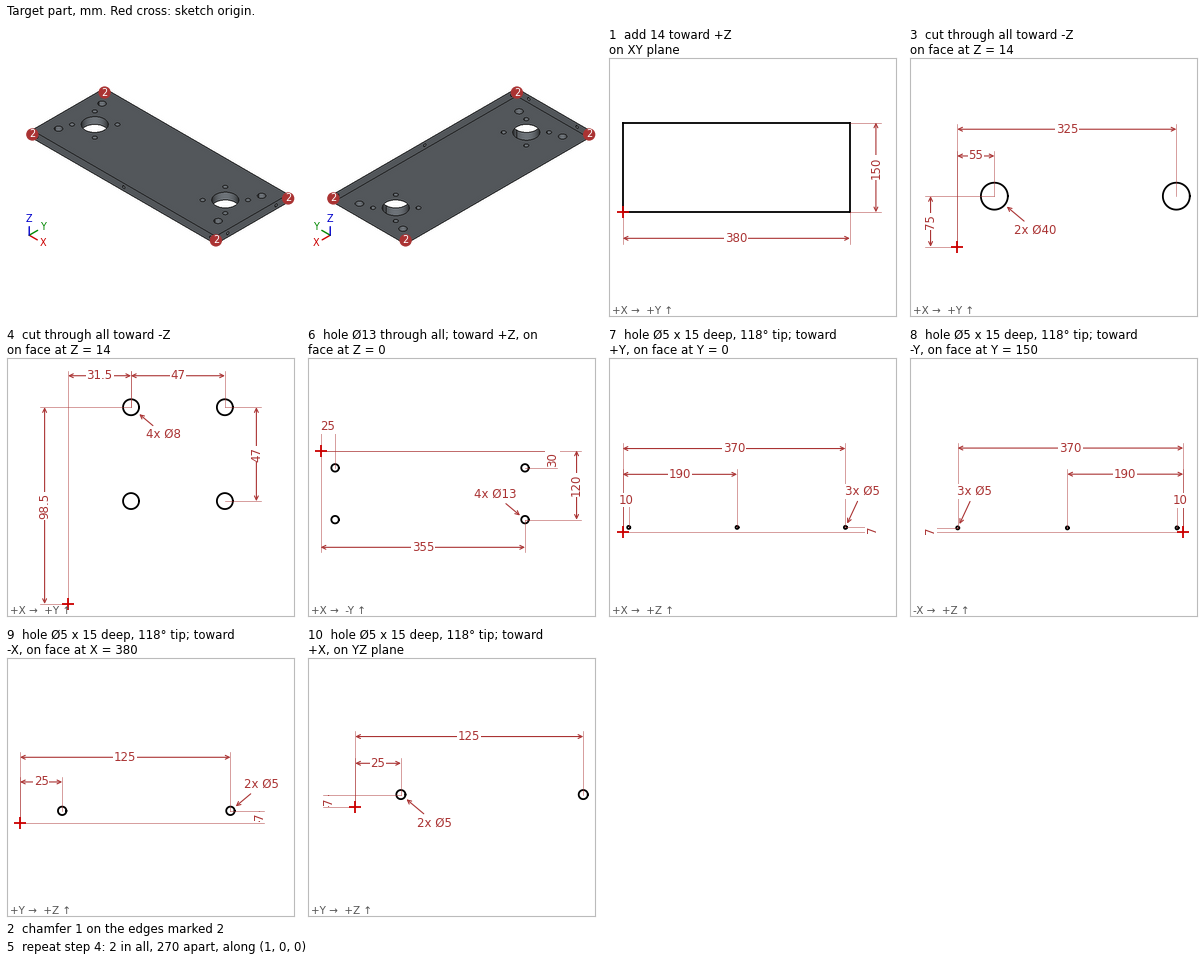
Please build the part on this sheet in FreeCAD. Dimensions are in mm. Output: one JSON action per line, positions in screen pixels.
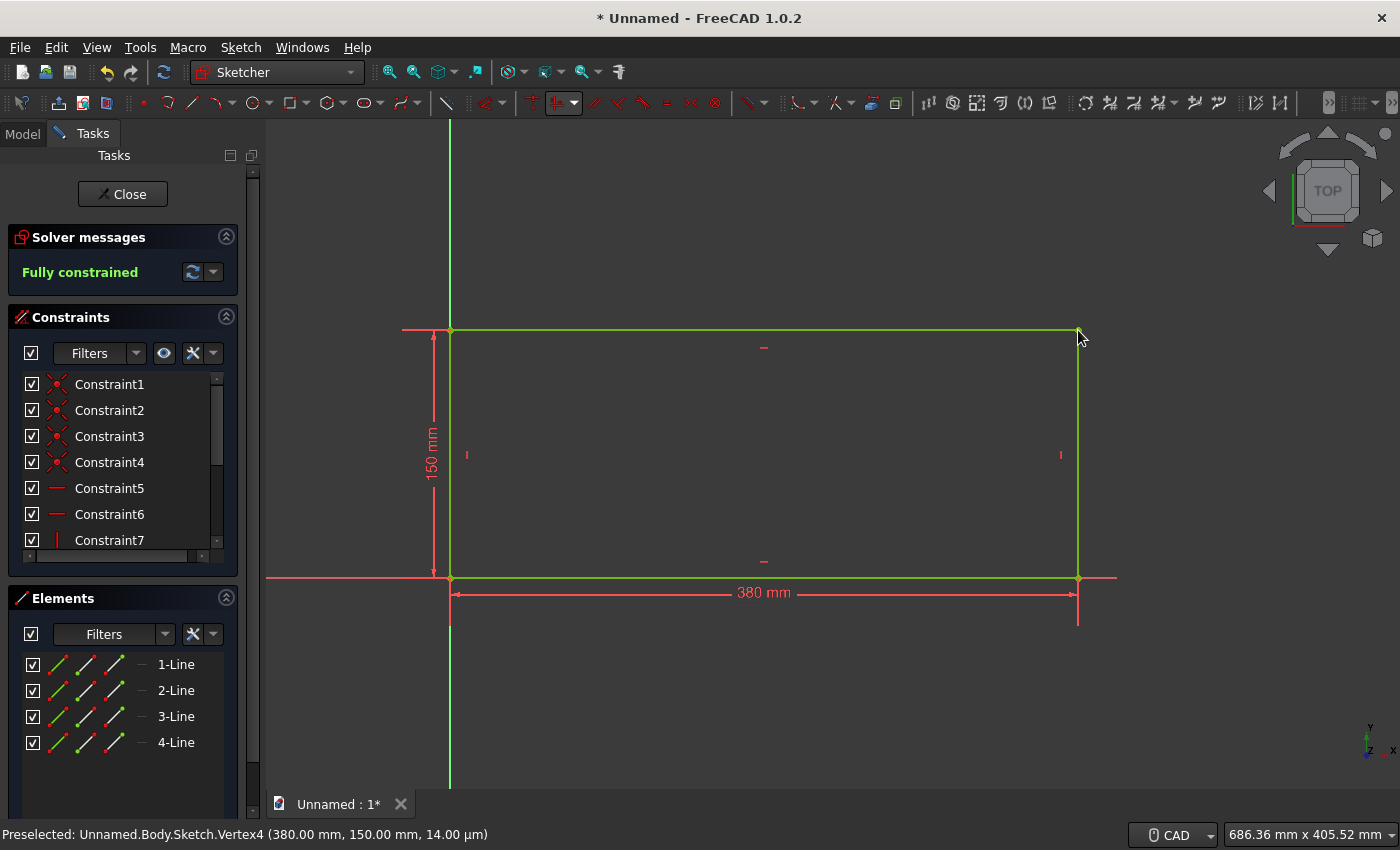
{"action": "left_click", "coordinate": [123, 194]}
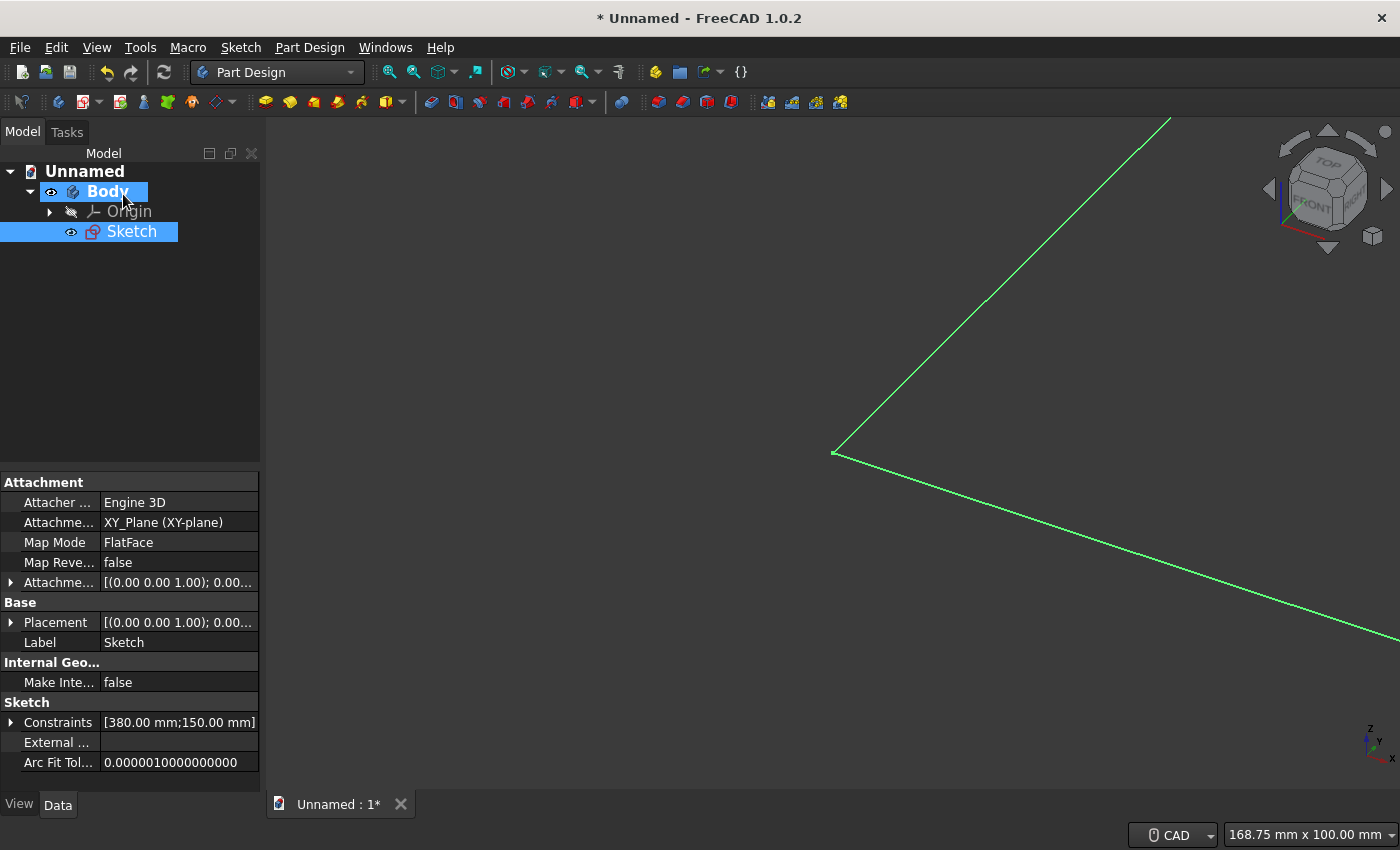
{"action": "left_click", "coordinate": [266, 102]}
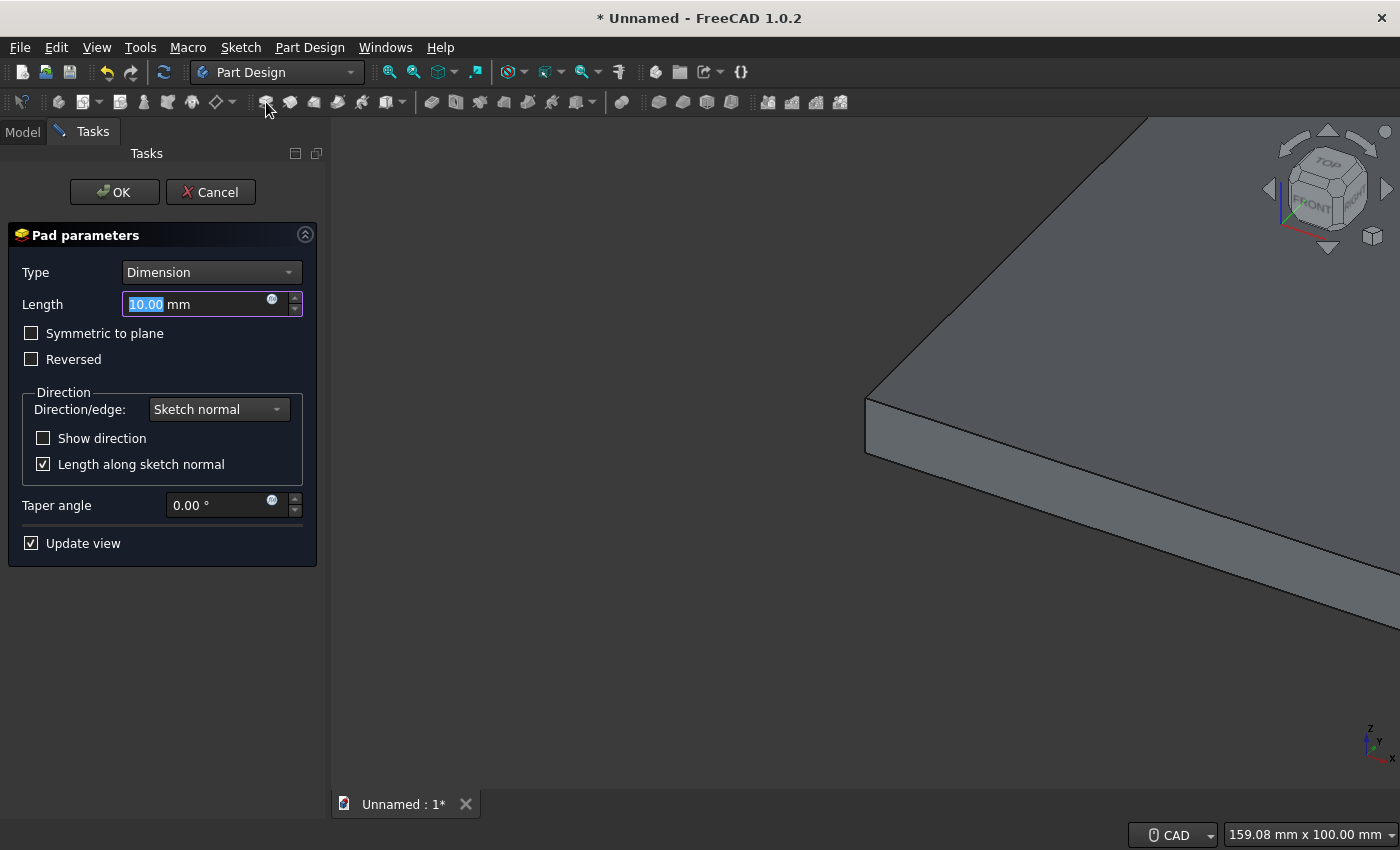
{"action": "type", "text": "14"}
{"action": "key", "text": "Tab"}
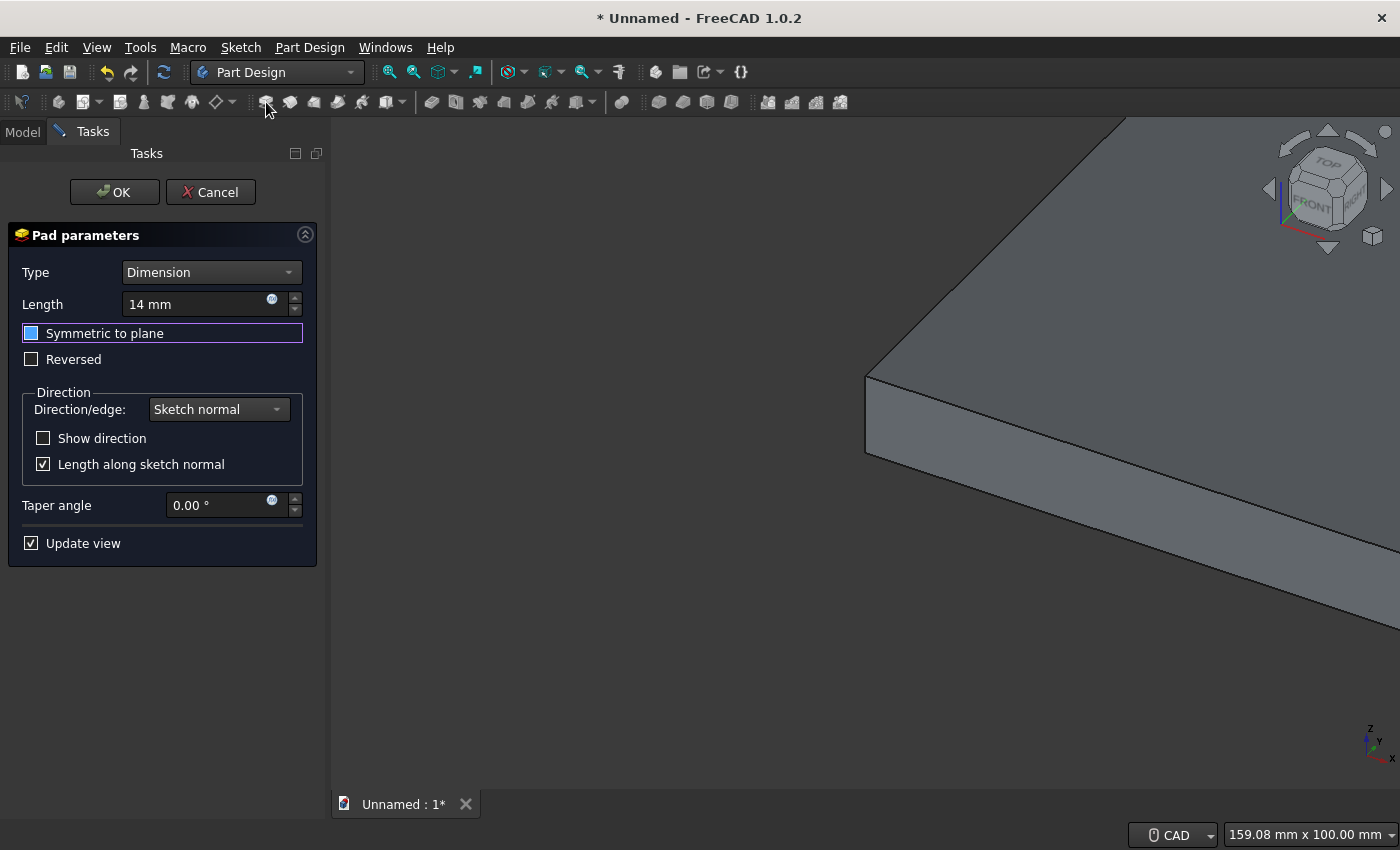
{"action": "left_click", "coordinate": [115, 192]}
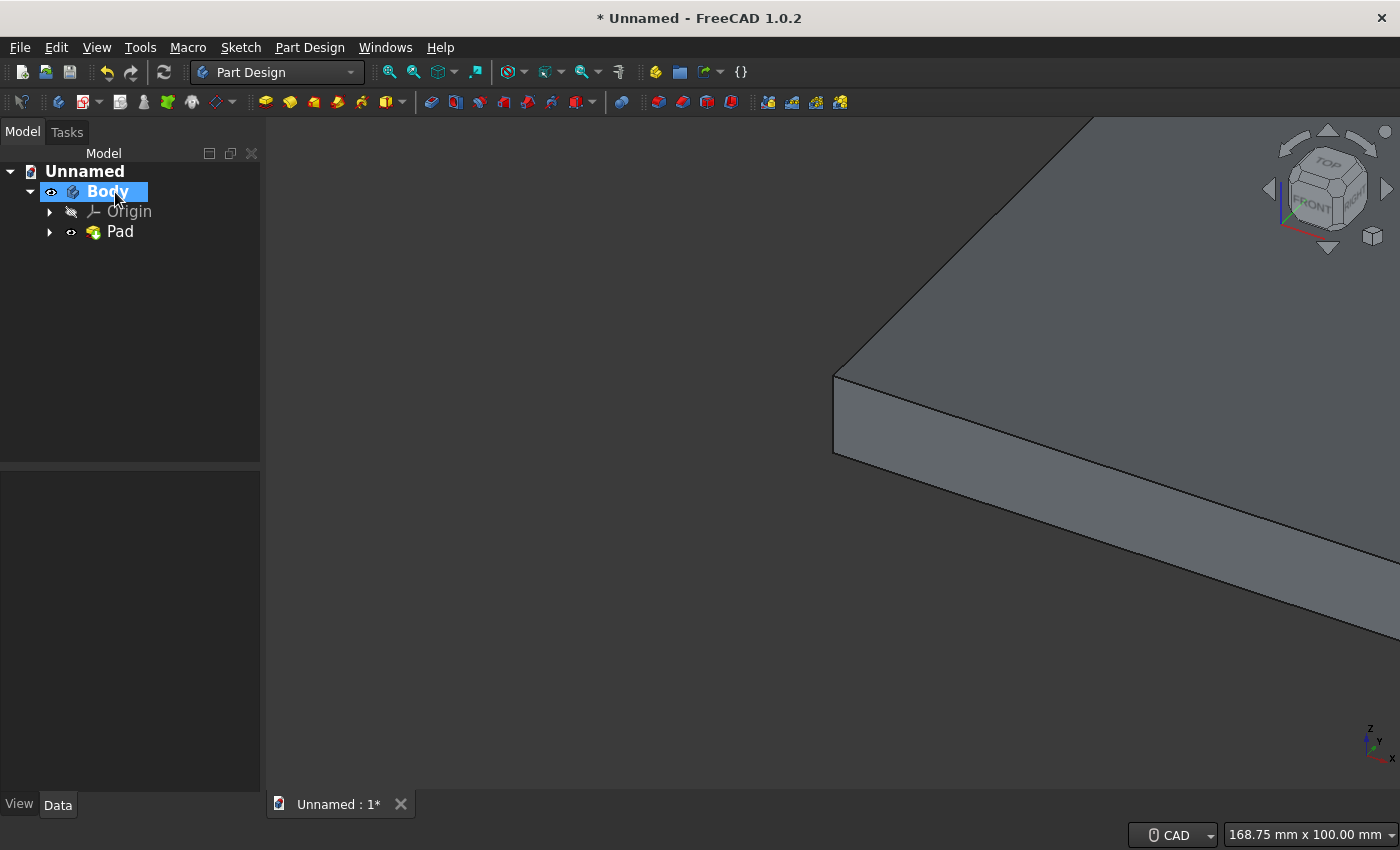
{"action": "key", "text": "v f"}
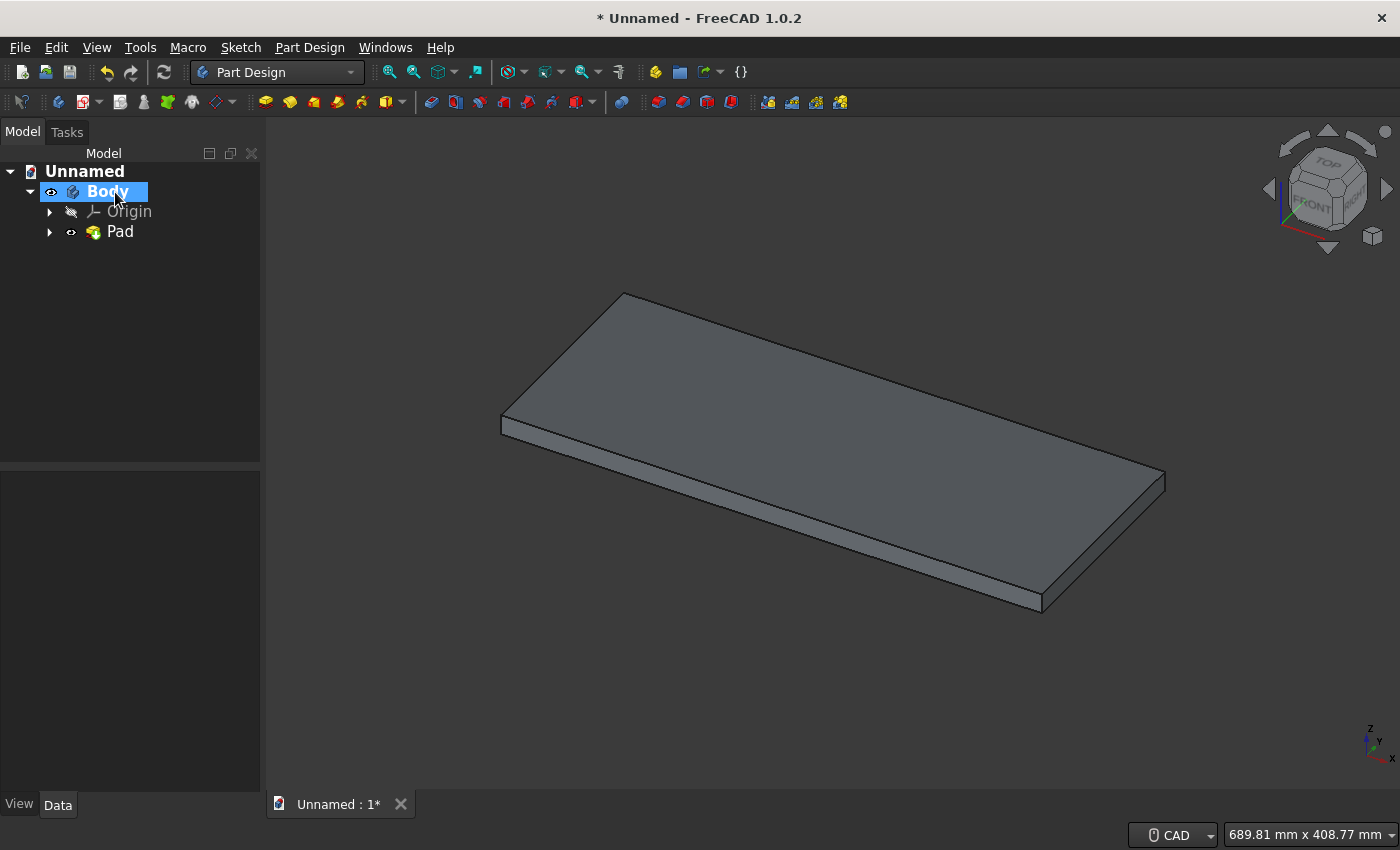
{"action": "left_click", "coordinate": [1042, 603]}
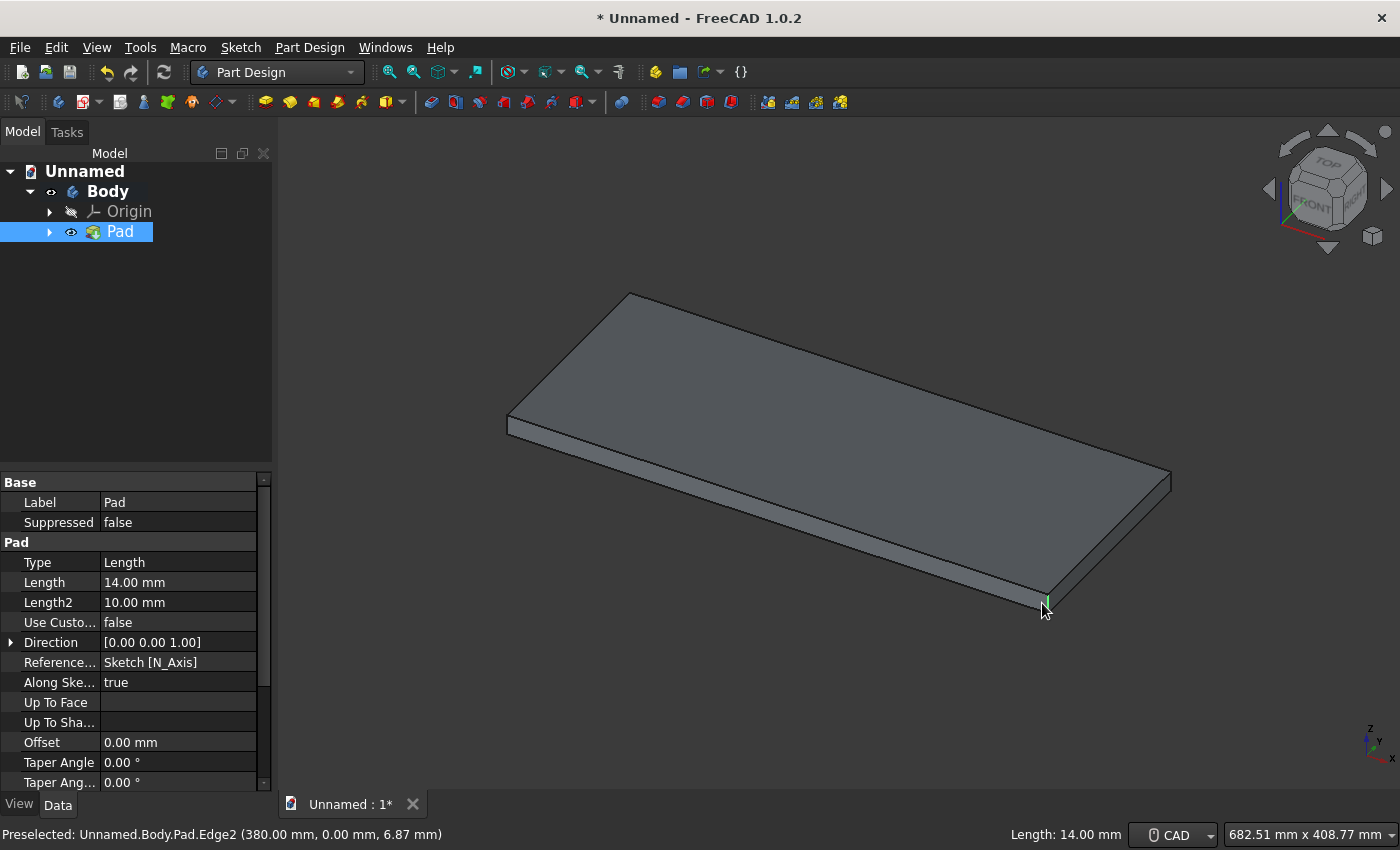
{"action": "key", "text": "0"}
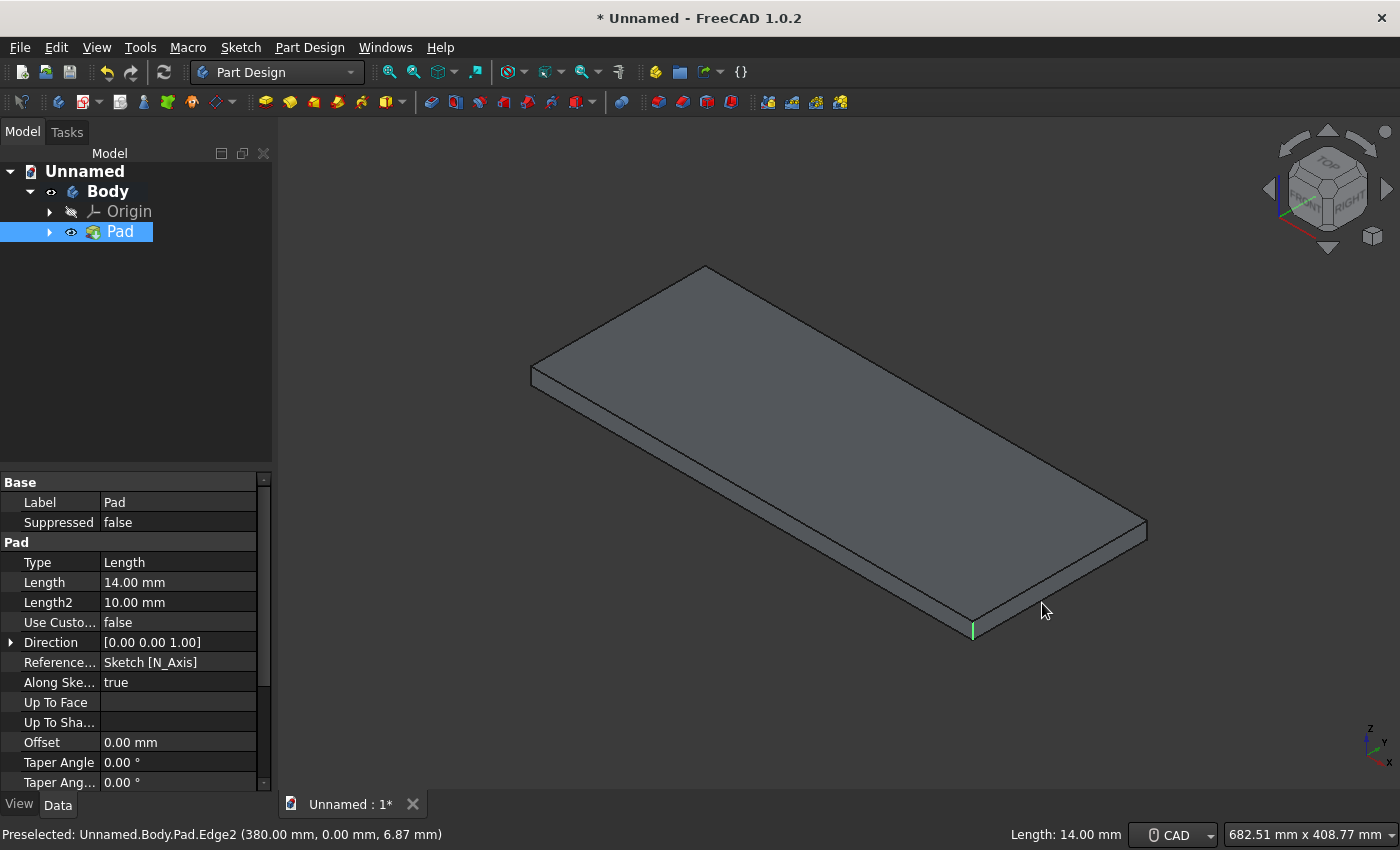
{"action": "key", "text": "2"}